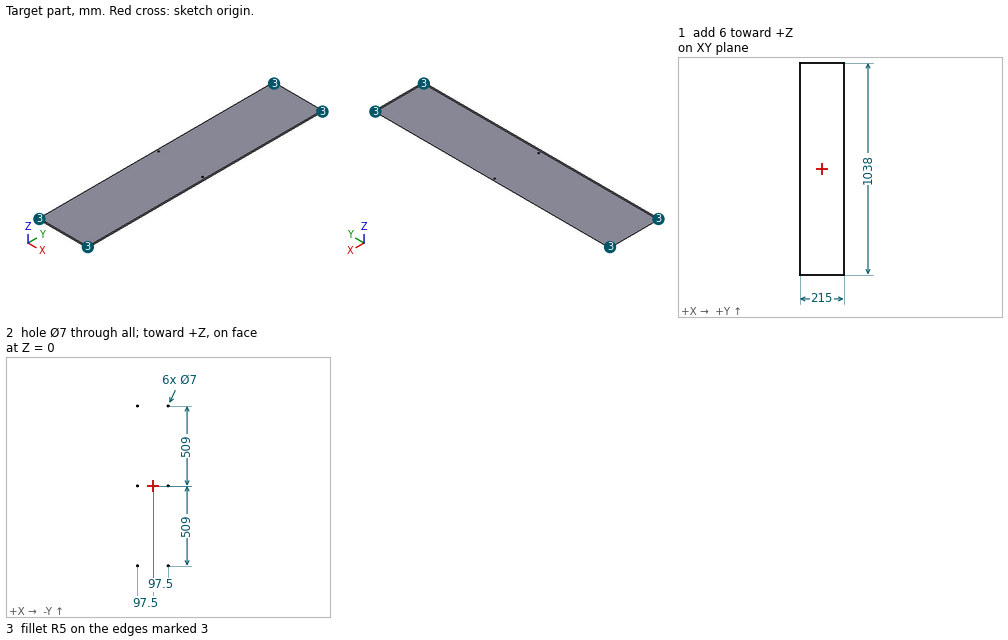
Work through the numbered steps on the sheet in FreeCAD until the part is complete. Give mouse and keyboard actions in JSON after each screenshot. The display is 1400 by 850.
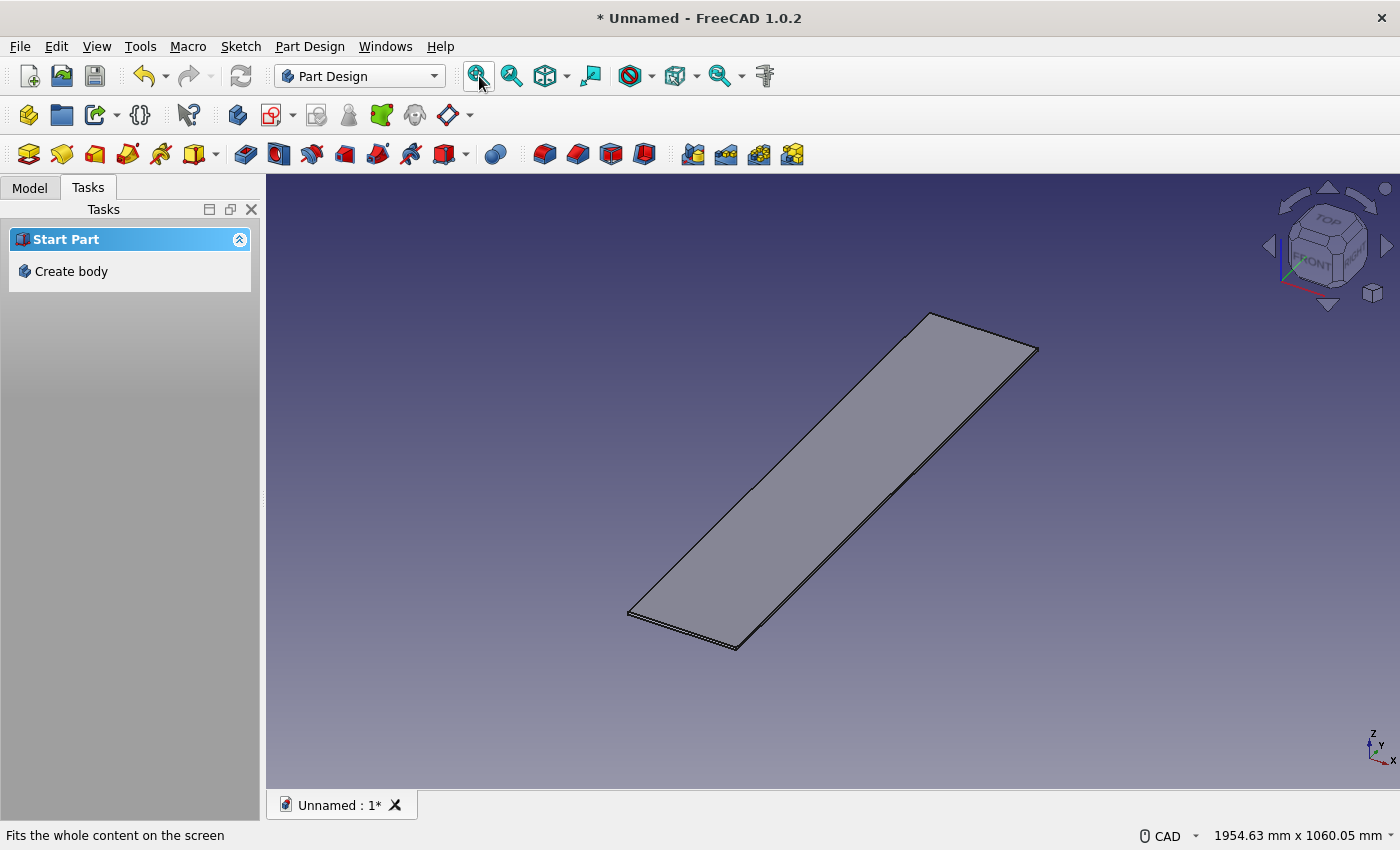
{"action": "key", "text": "5"}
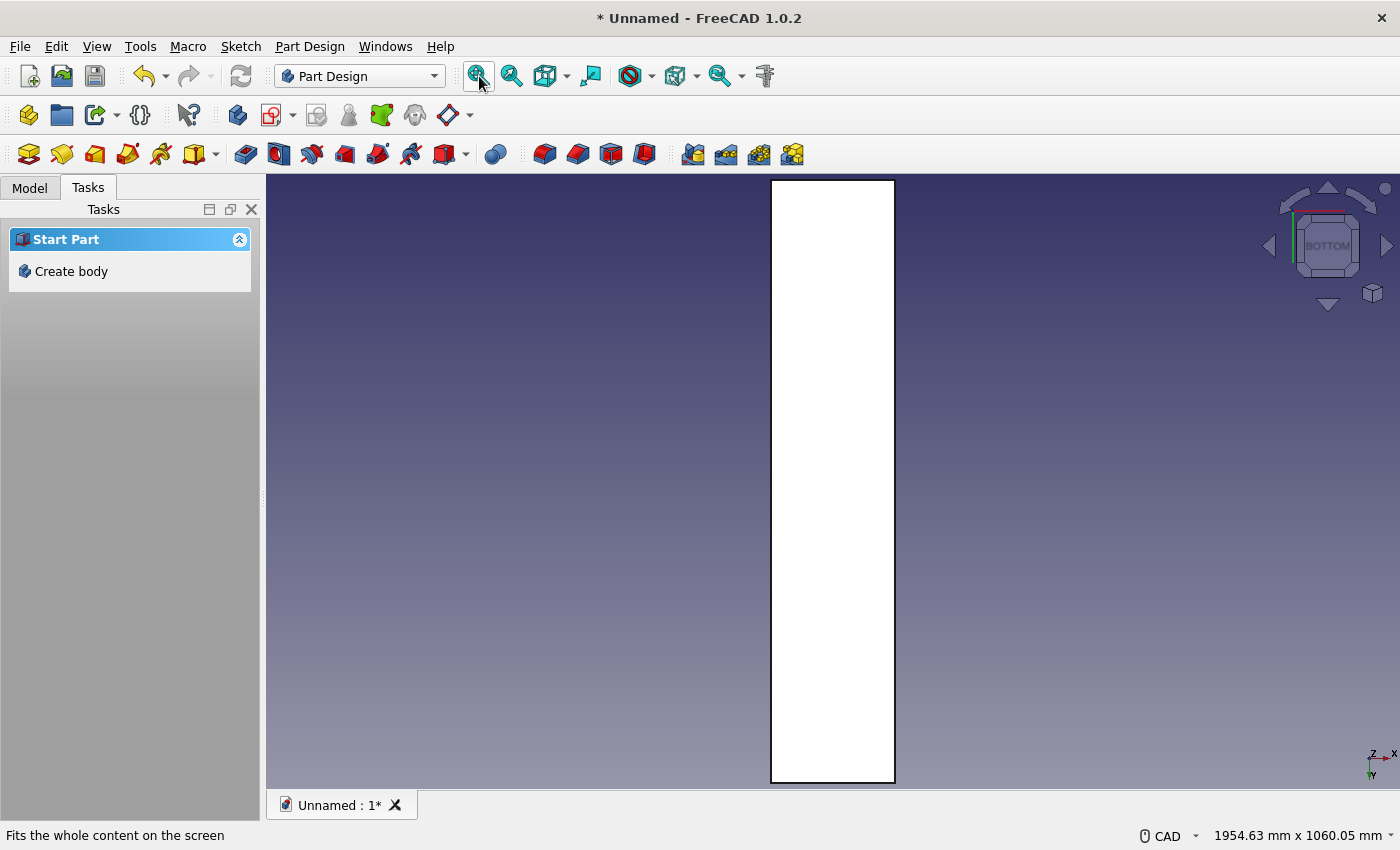
{"action": "left_click", "coordinate": [833, 653]}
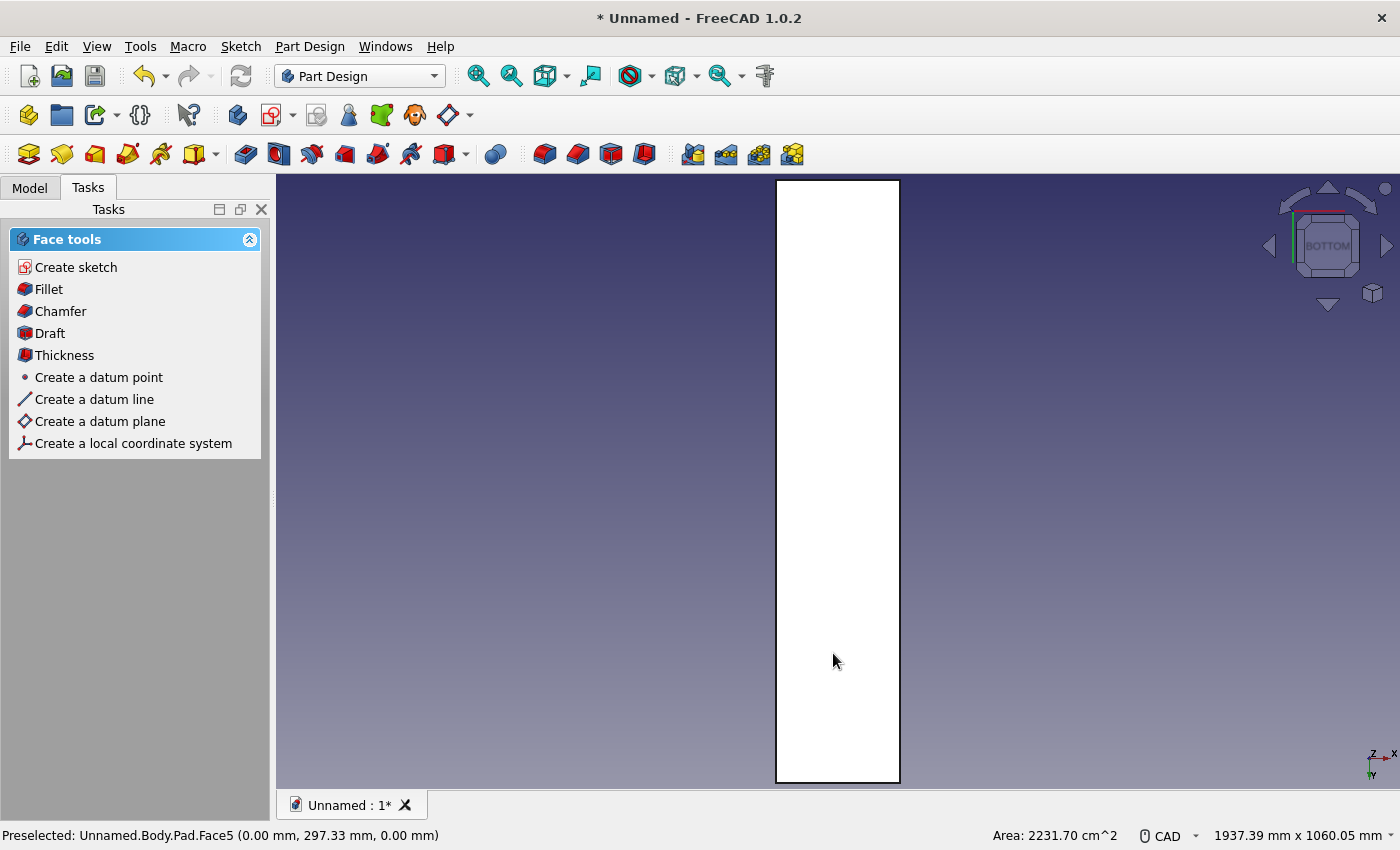
{"action": "left_click", "coordinate": [270, 116]}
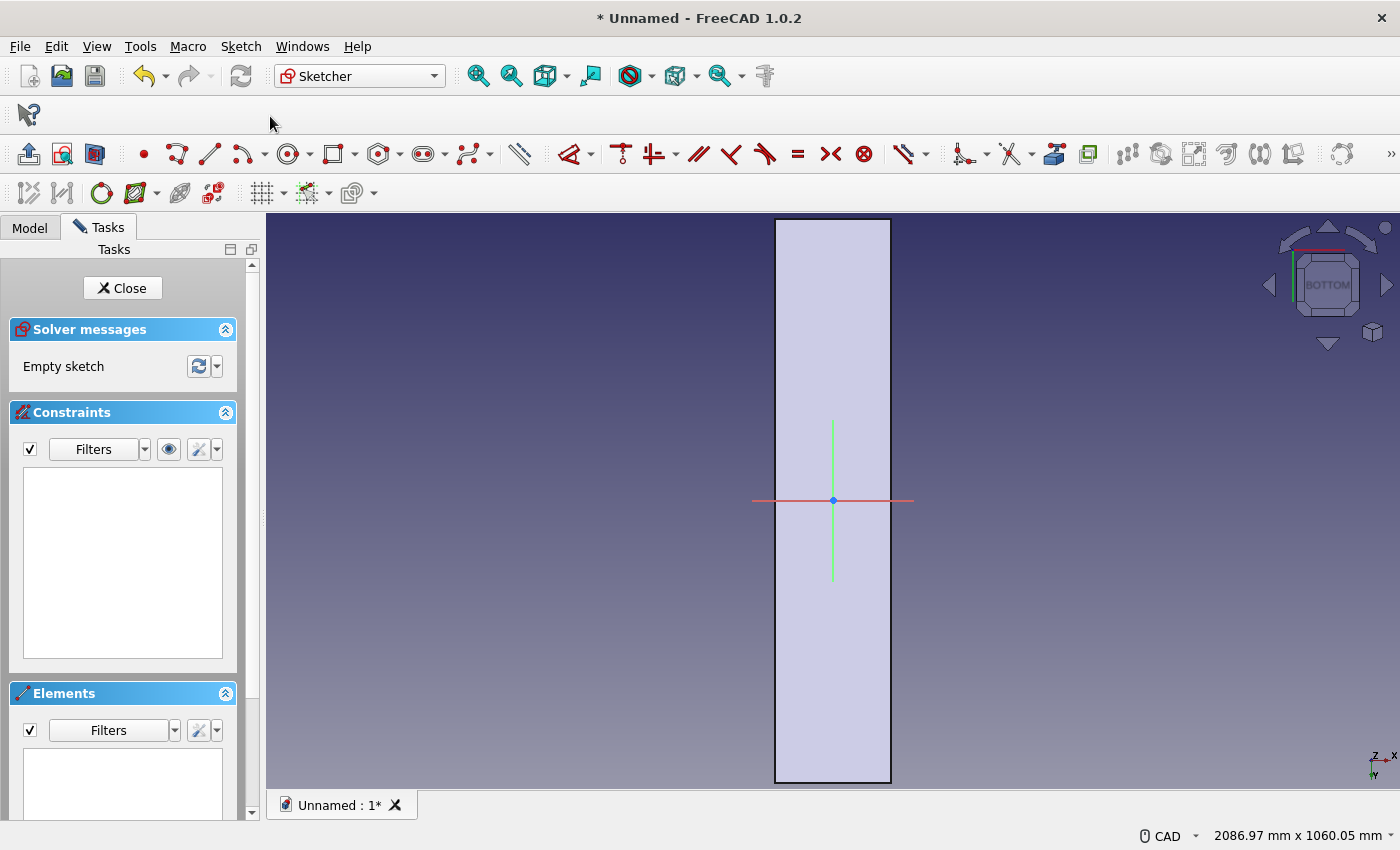
{"action": "scroll", "coordinate": [625, 501], "scroll_direction": "down", "scroll_amount": 2}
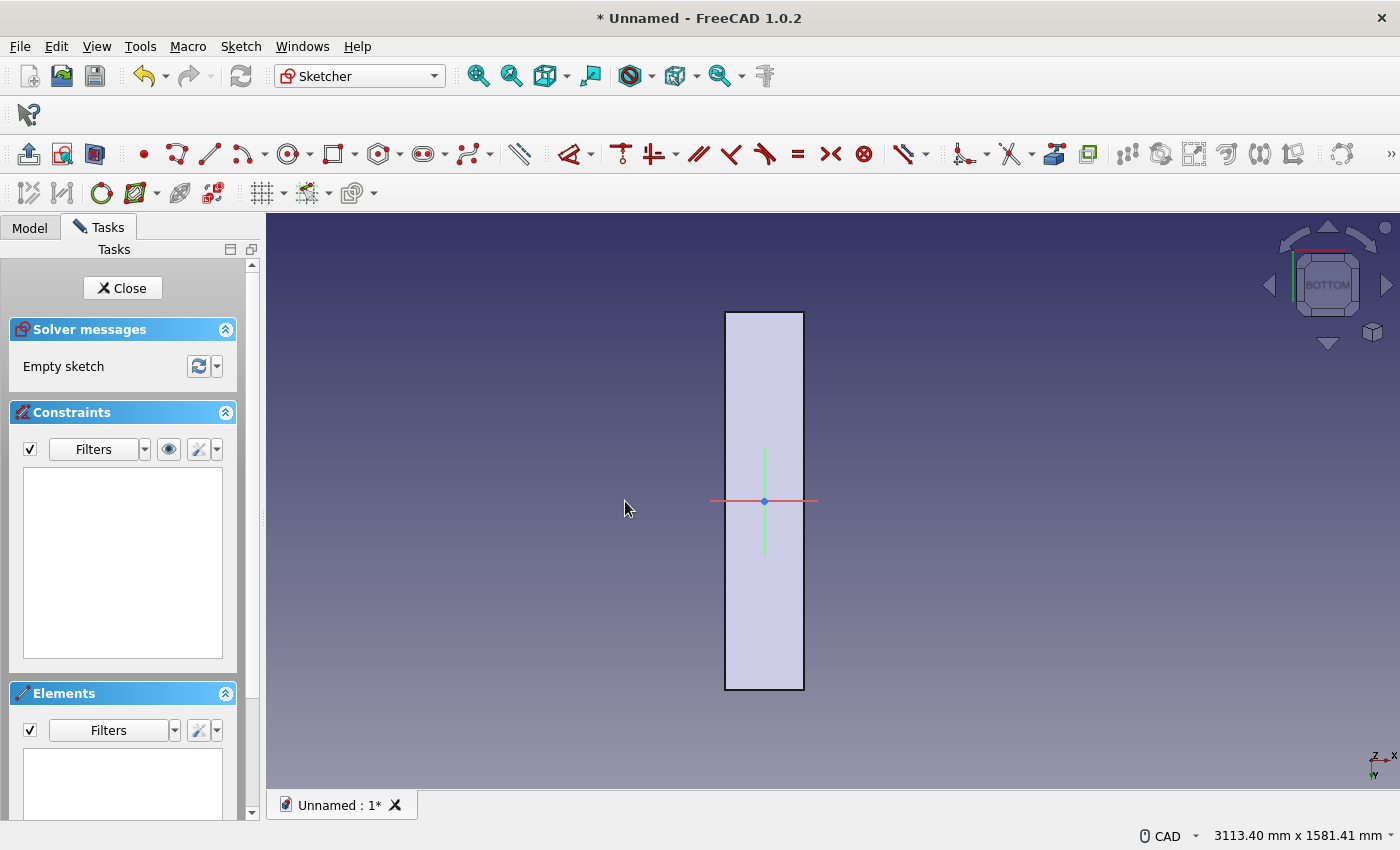
{"action": "key", "text": "g c"}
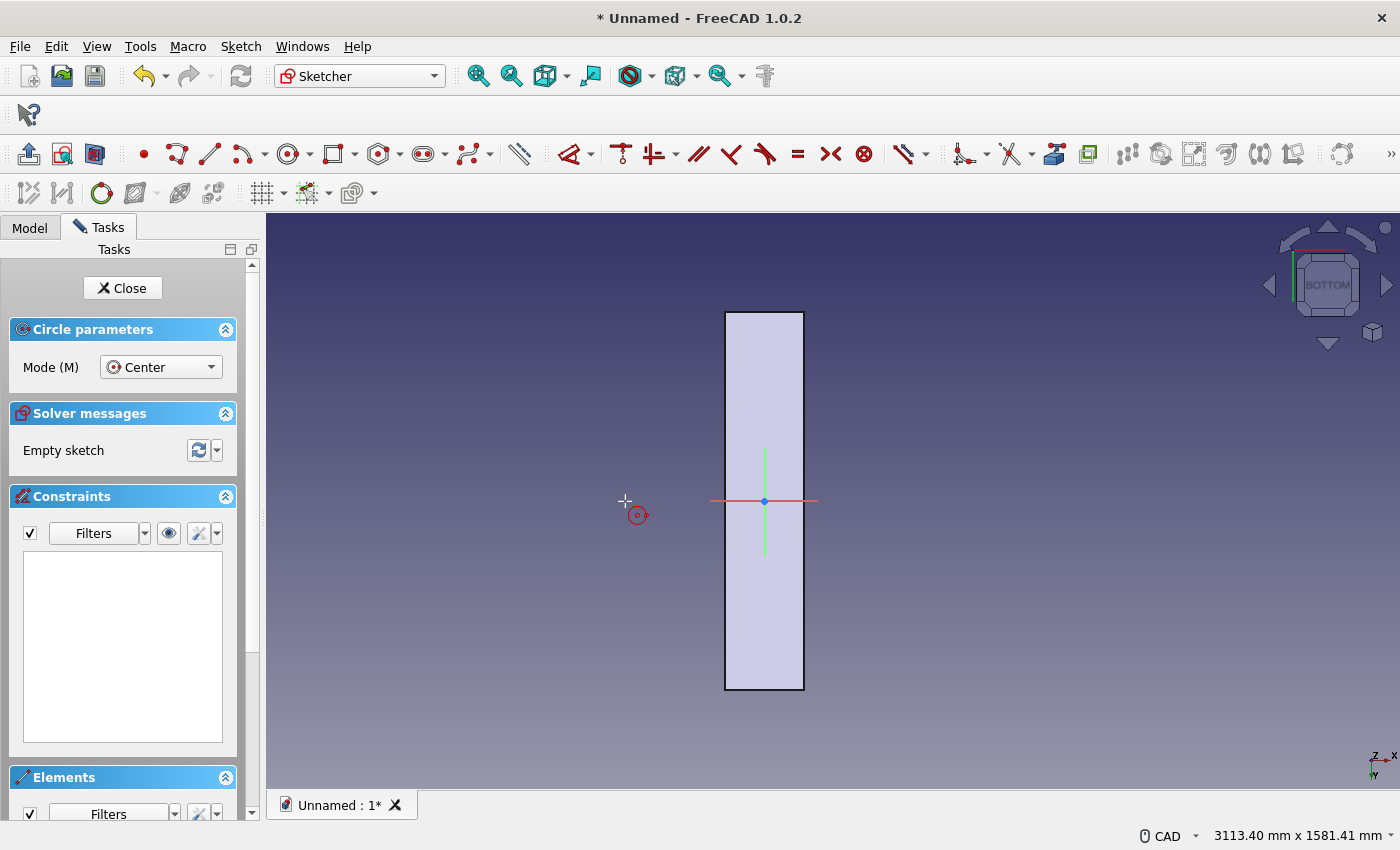
{"action": "scroll", "coordinate": [800, 687], "scroll_direction": "up", "scroll_amount": 15}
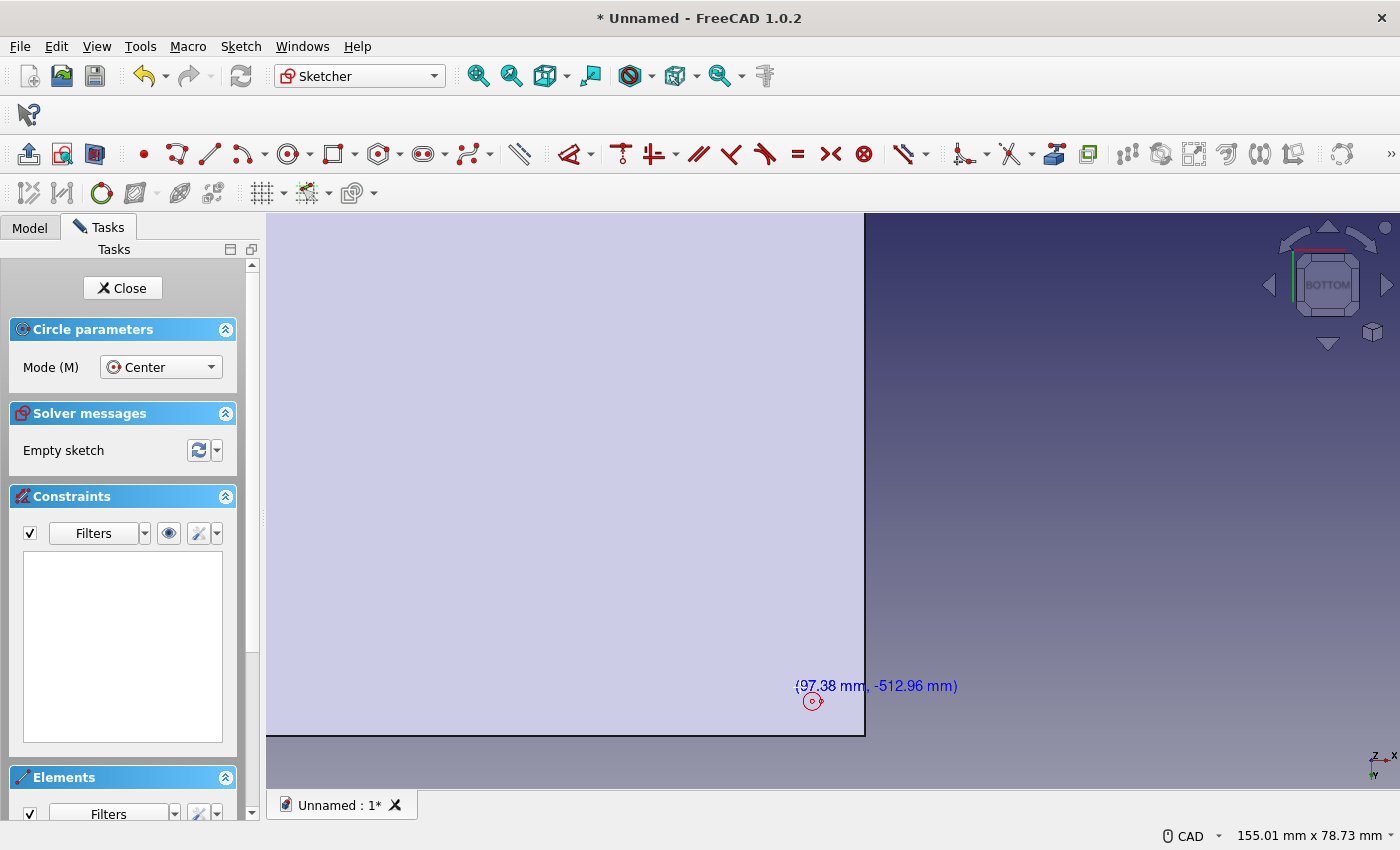
{"action": "scroll", "coordinate": [800, 688], "scroll_direction": "down", "scroll_amount": 15}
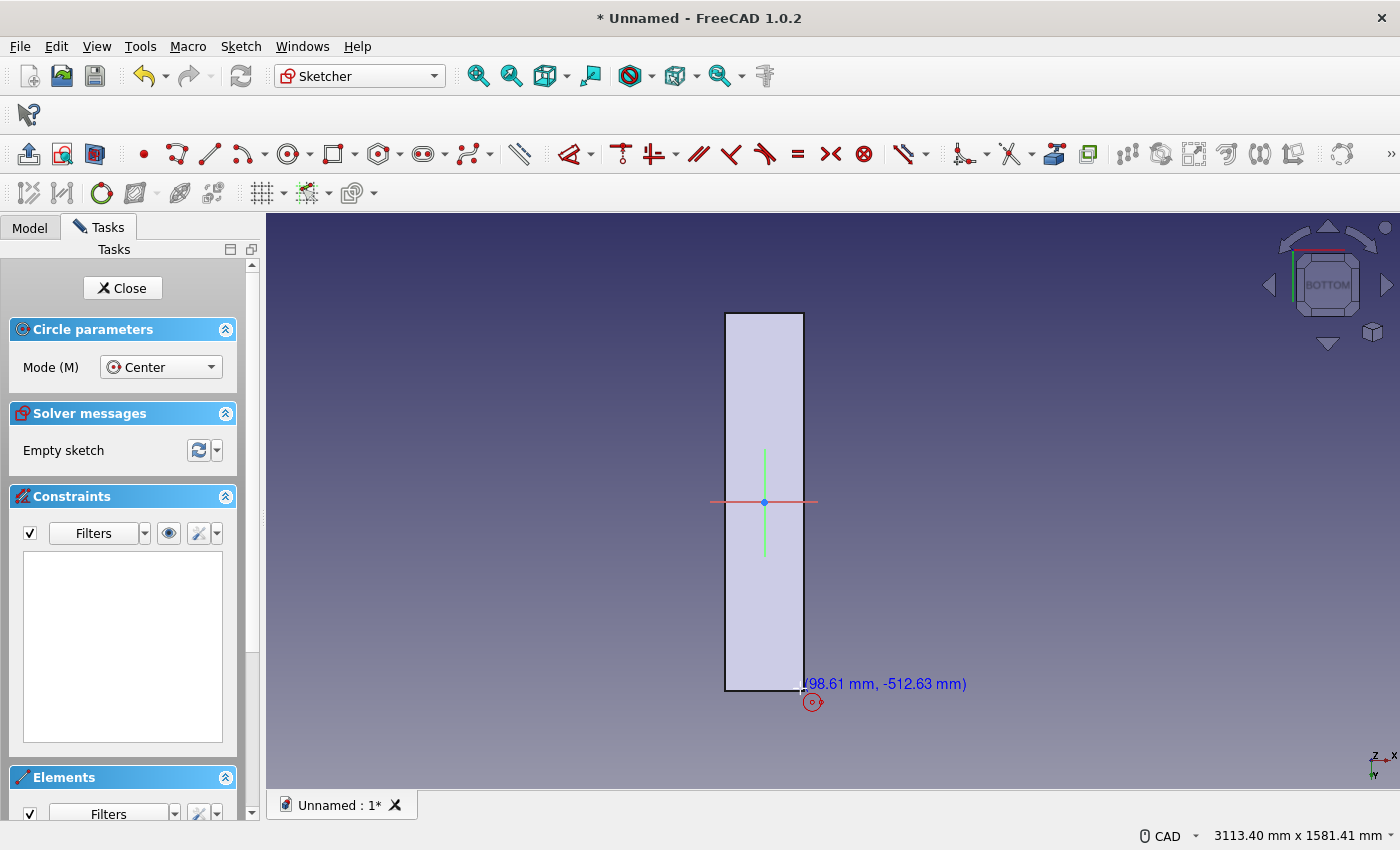
{"action": "left_click", "coordinate": [800, 688]}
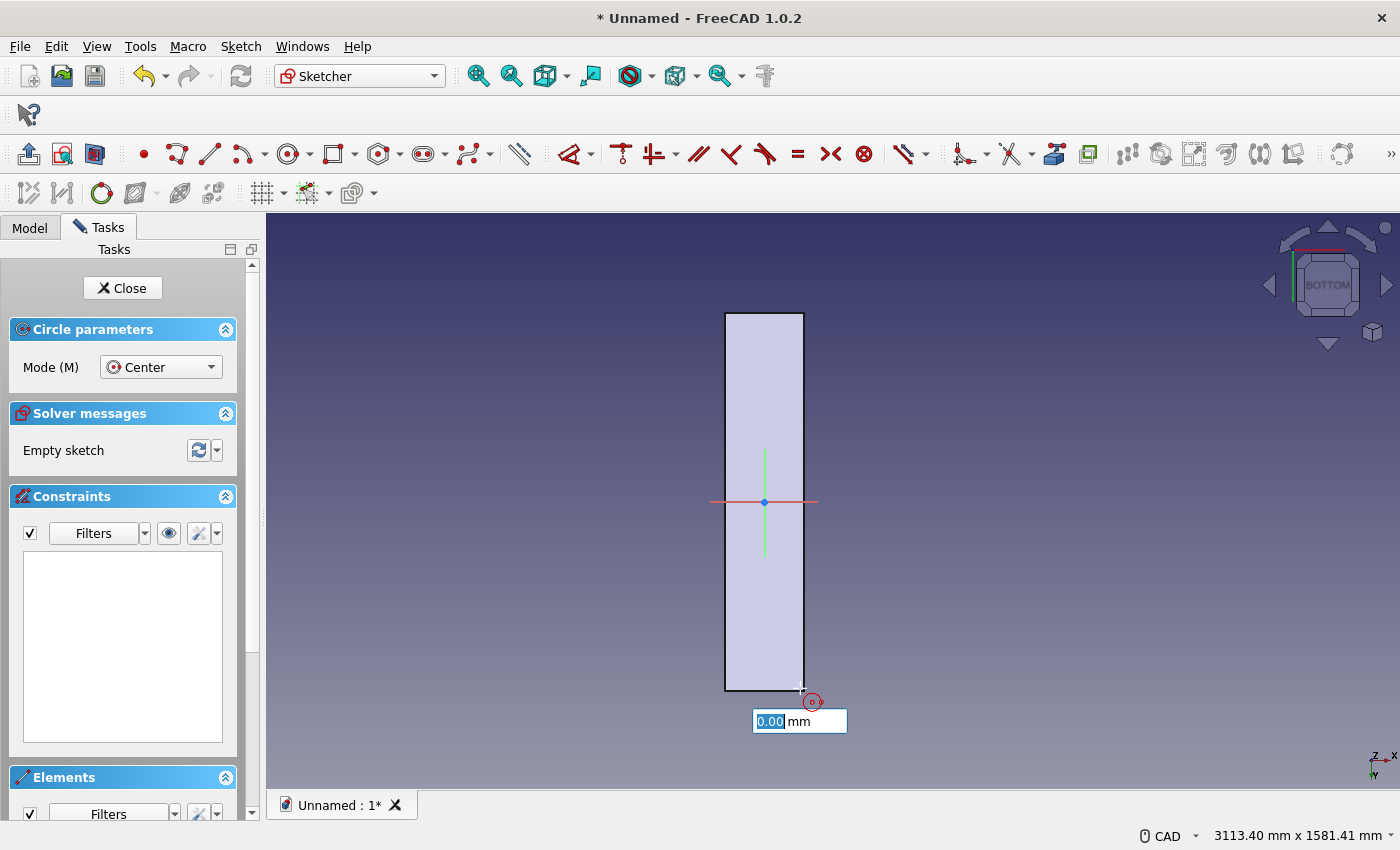
{"action": "scroll", "coordinate": [801, 687], "scroll_direction": "up", "scroll_amount": 13}